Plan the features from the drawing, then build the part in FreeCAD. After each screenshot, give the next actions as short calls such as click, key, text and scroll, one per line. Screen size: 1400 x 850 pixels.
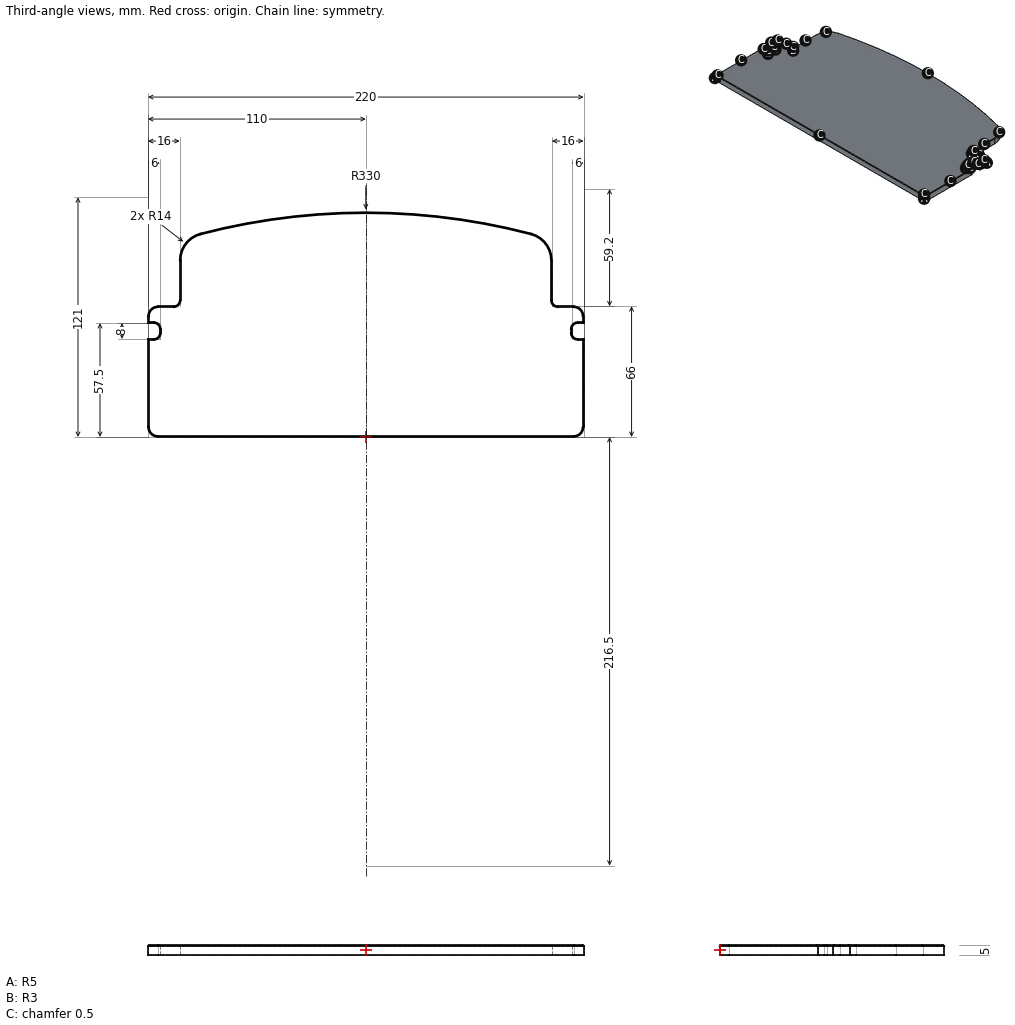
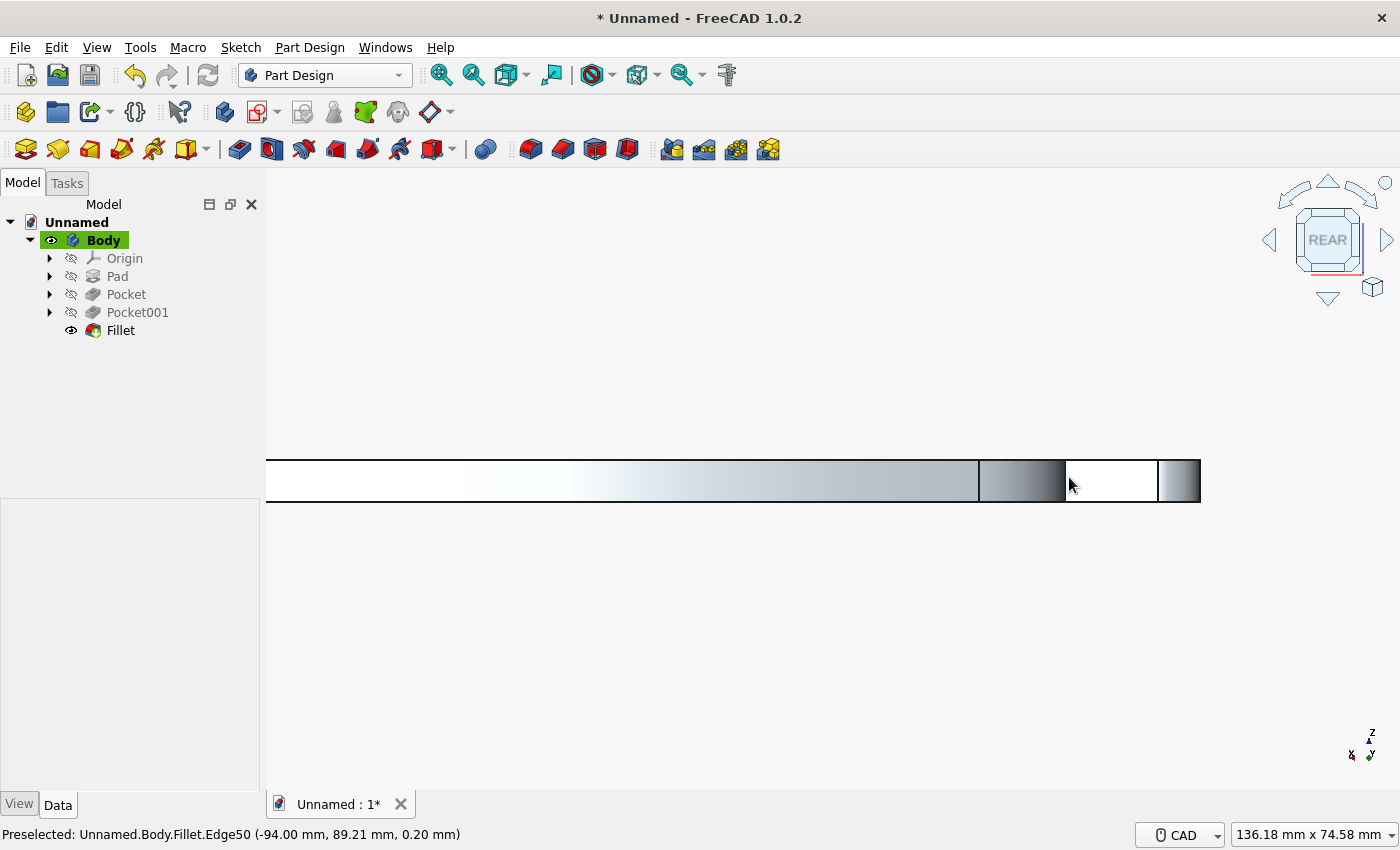
key(v)
key(f)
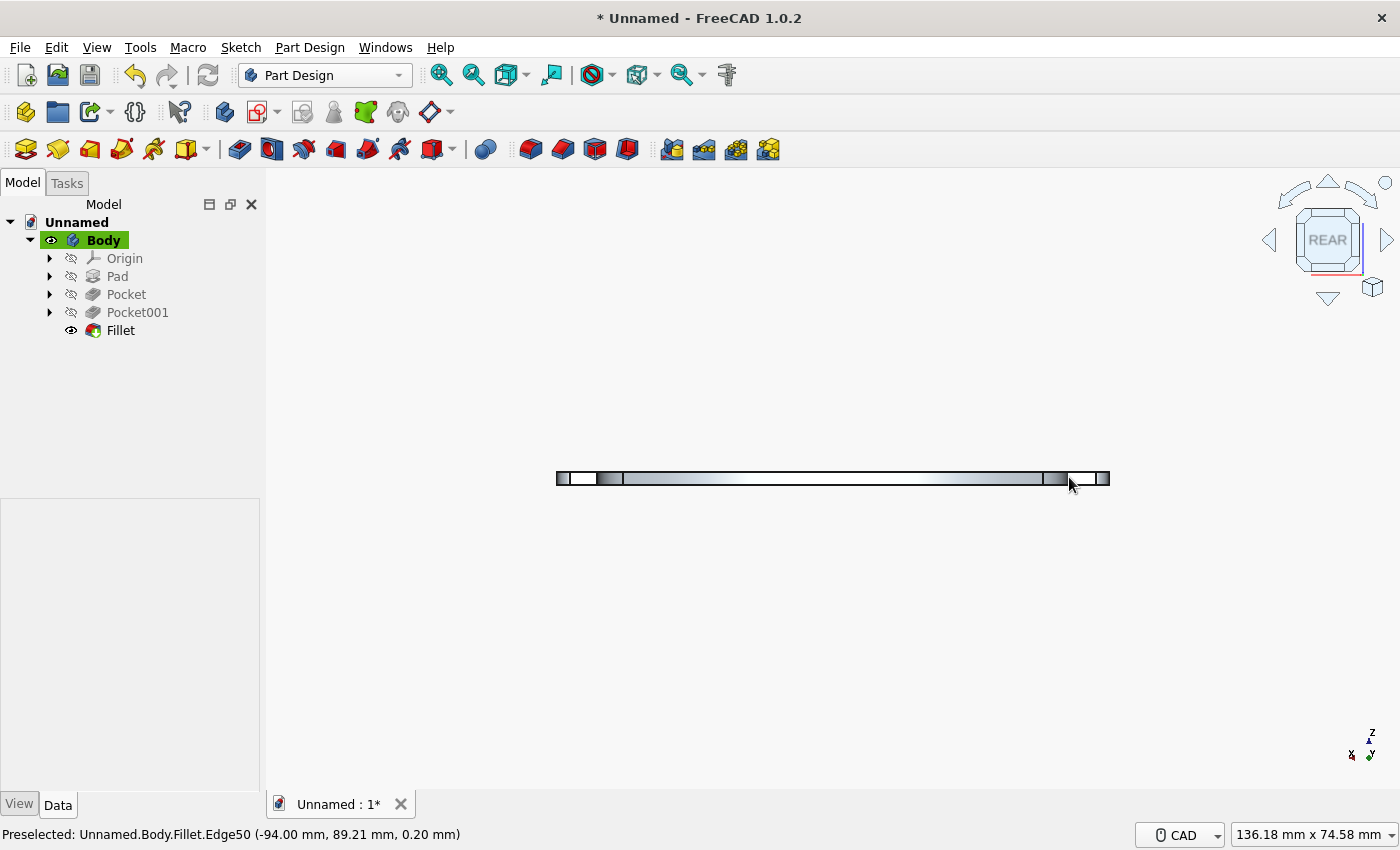
key(6)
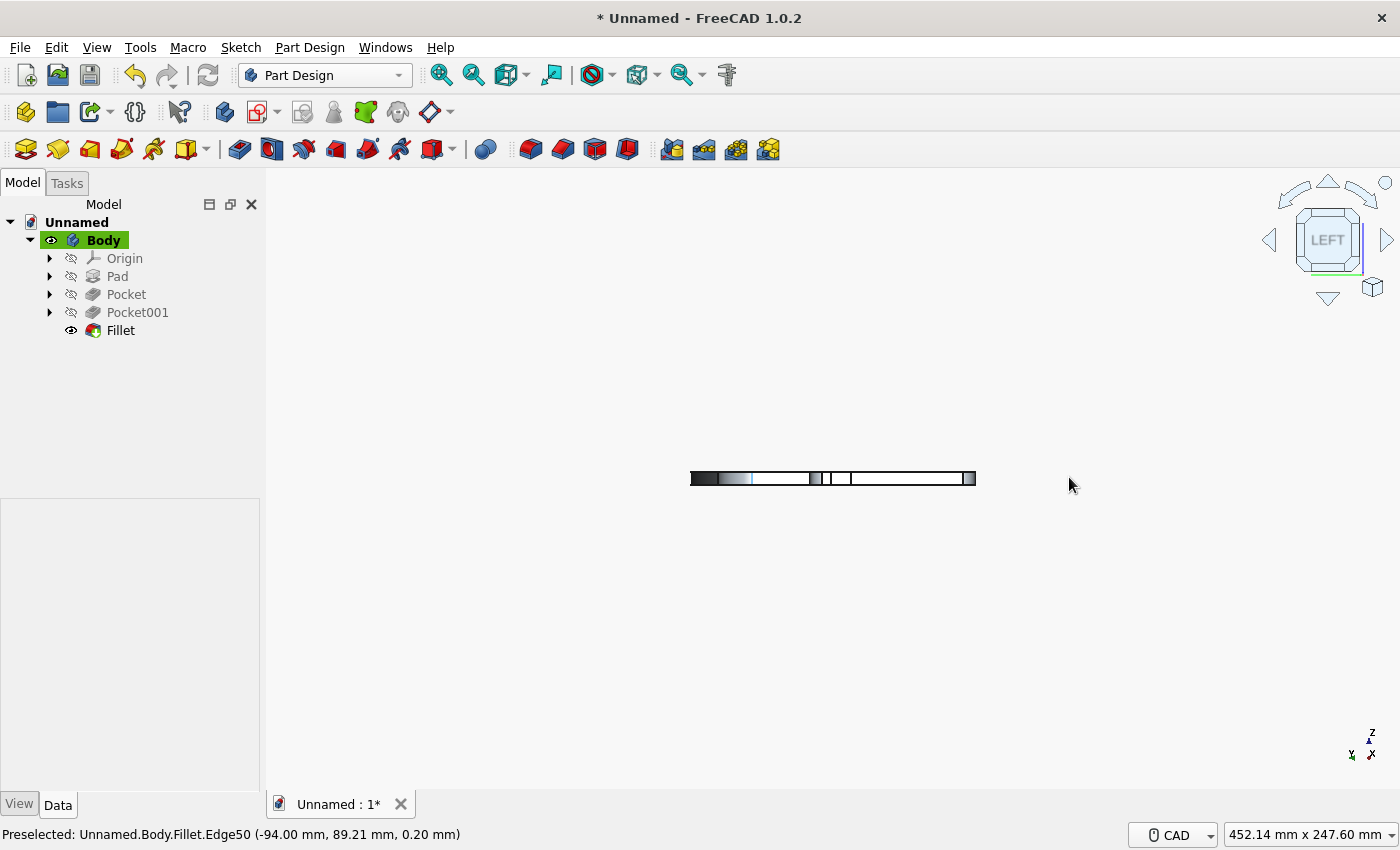
key(v)
key(f)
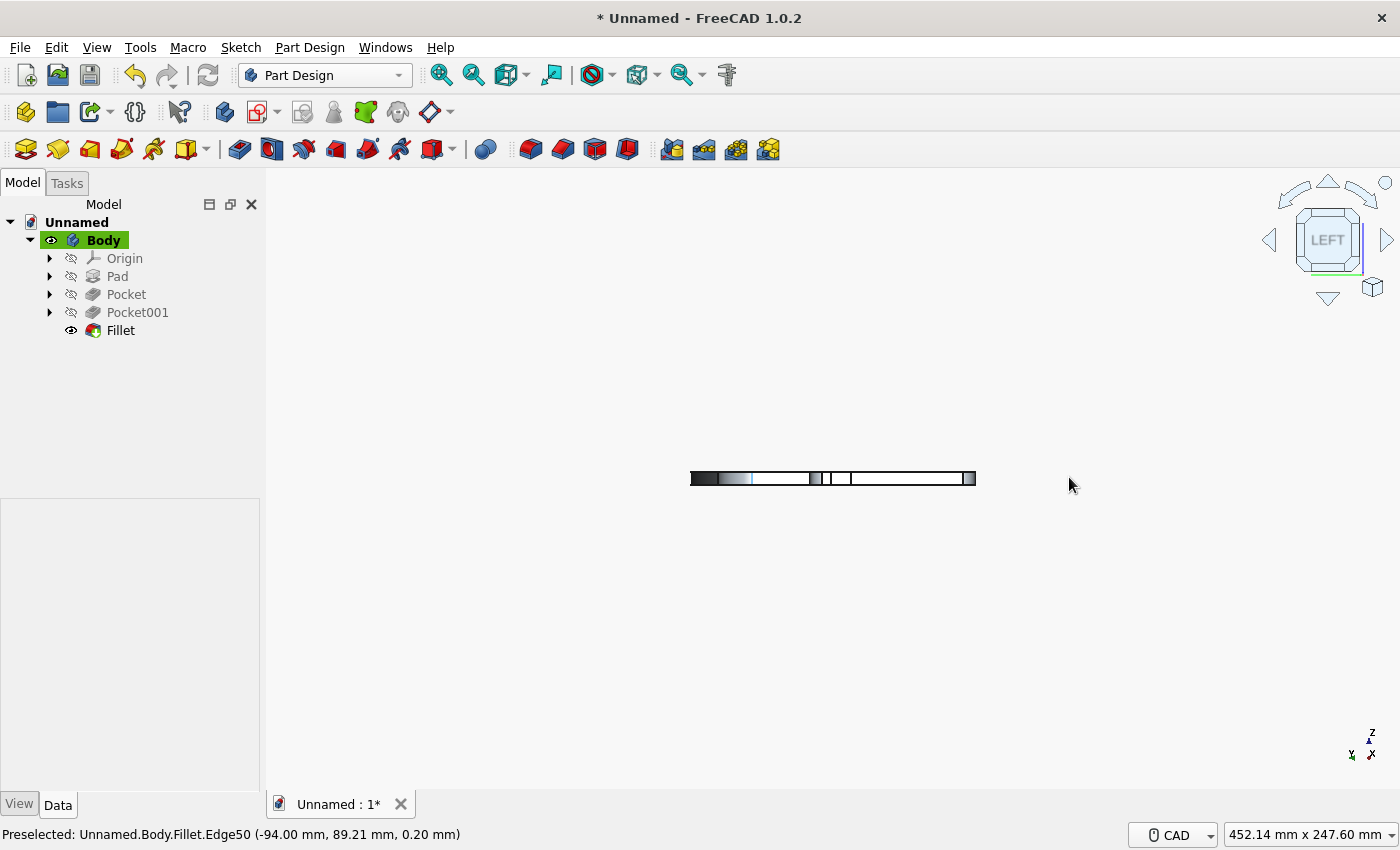
scroll(810, 477, up, 6)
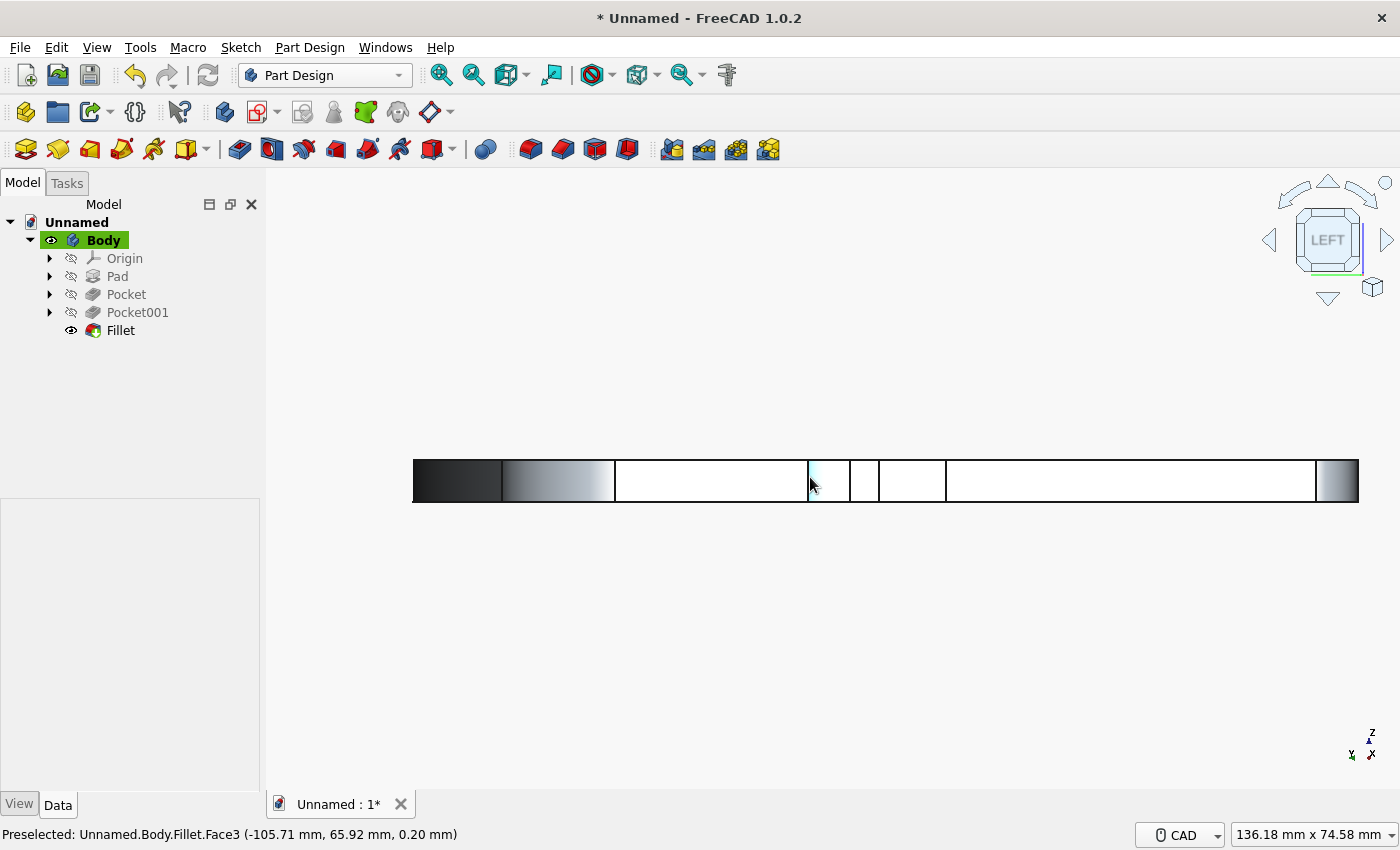
key(v)
key(f)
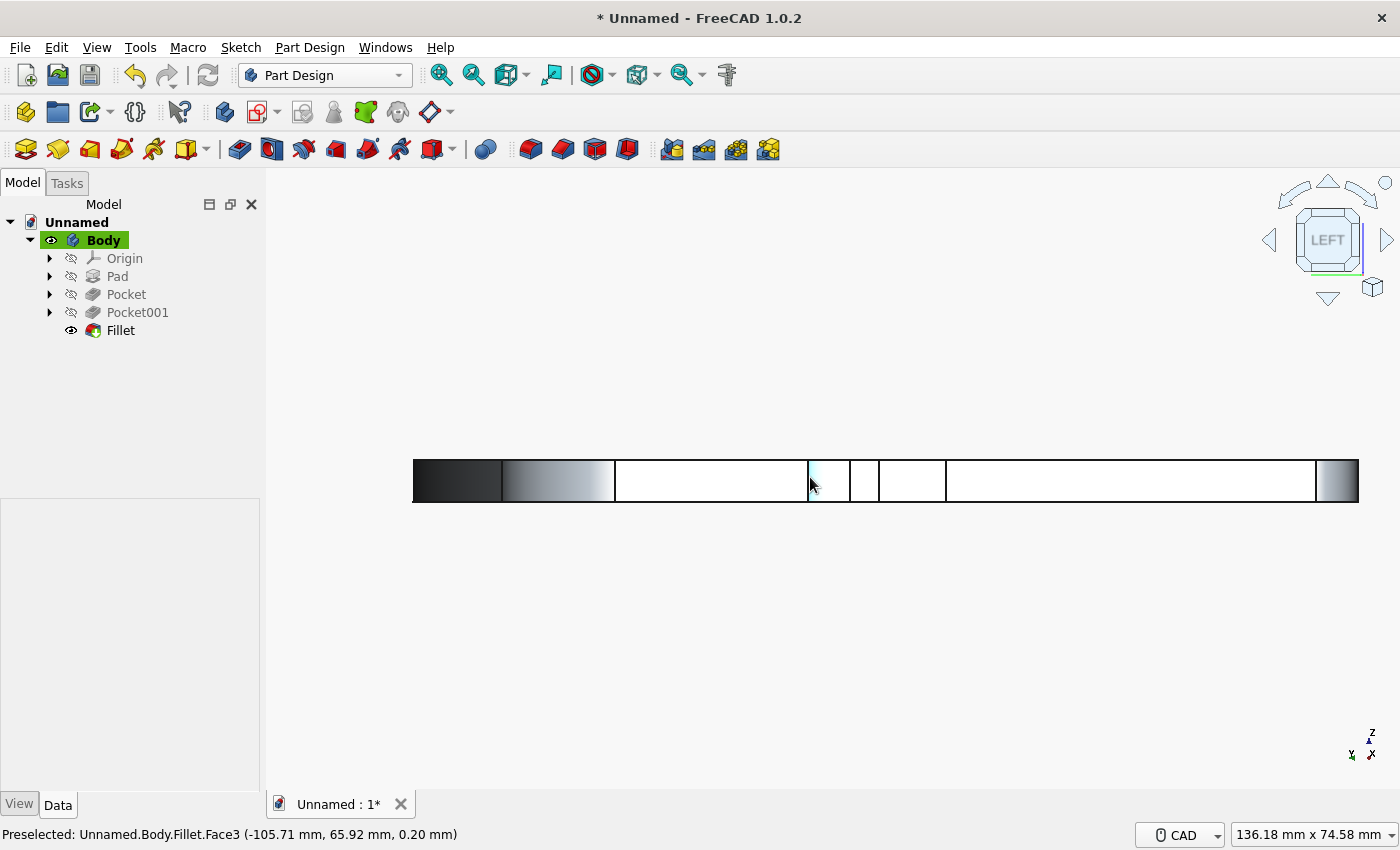
key(v)
key(3)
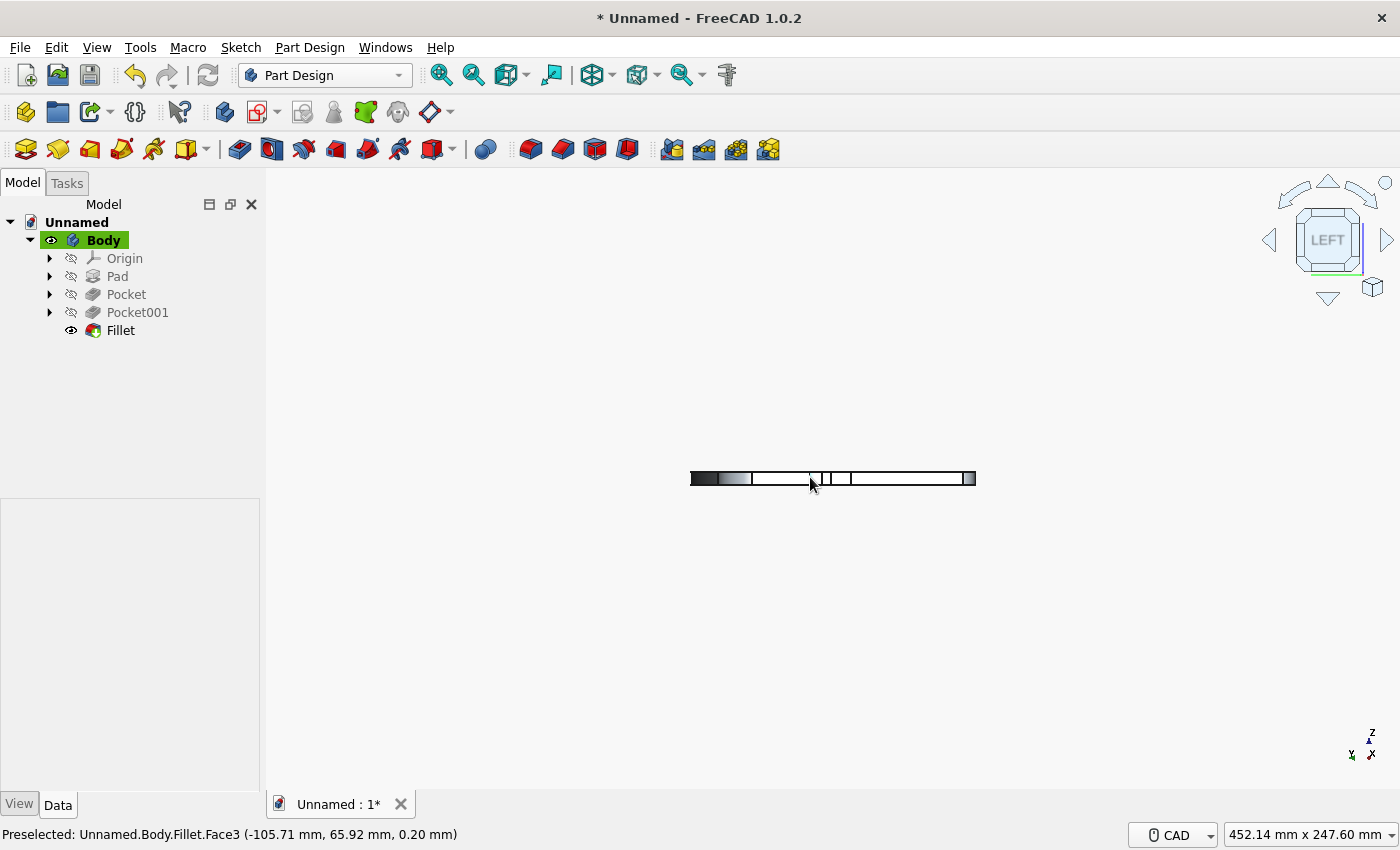
key(0)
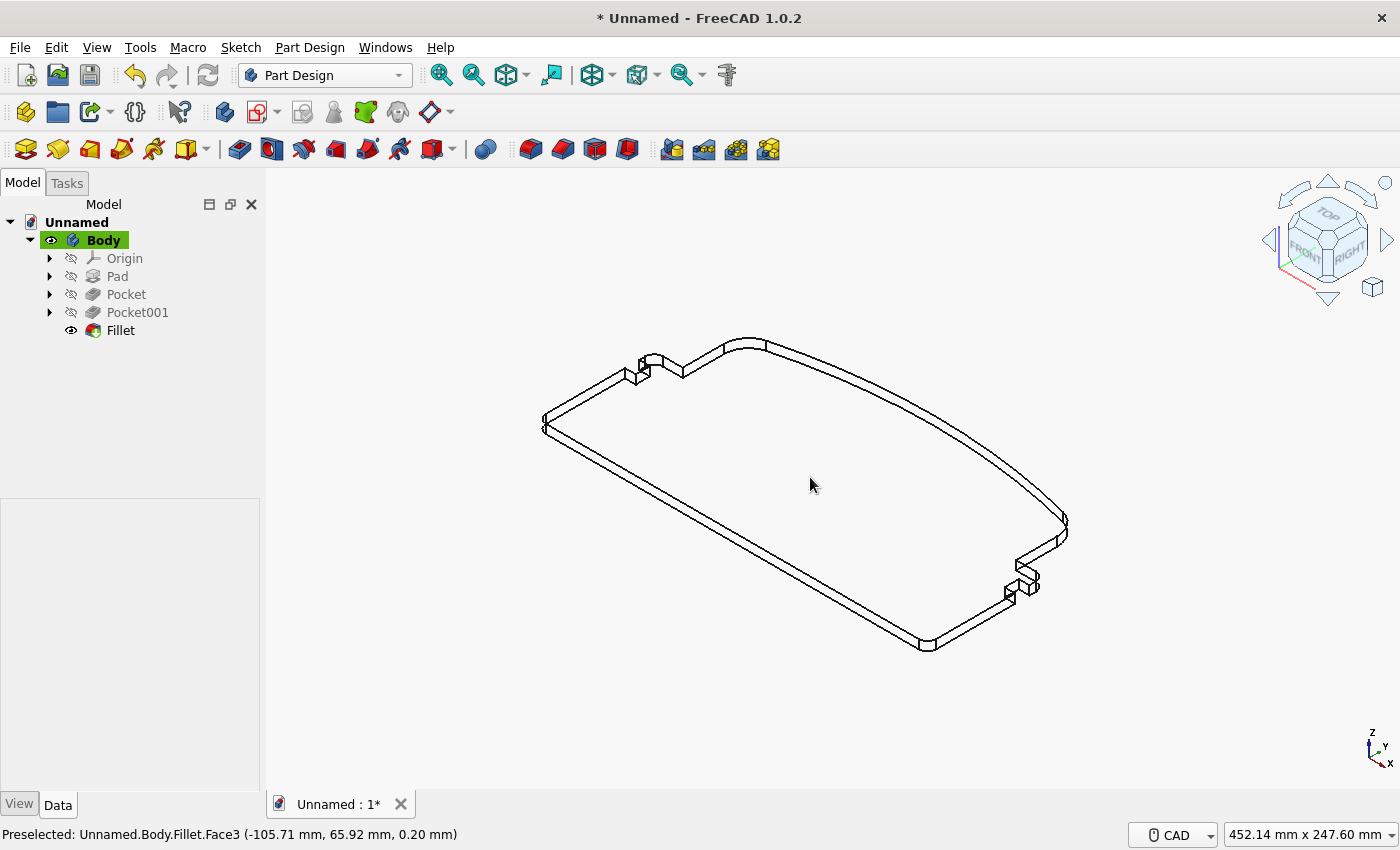
click(683, 373)